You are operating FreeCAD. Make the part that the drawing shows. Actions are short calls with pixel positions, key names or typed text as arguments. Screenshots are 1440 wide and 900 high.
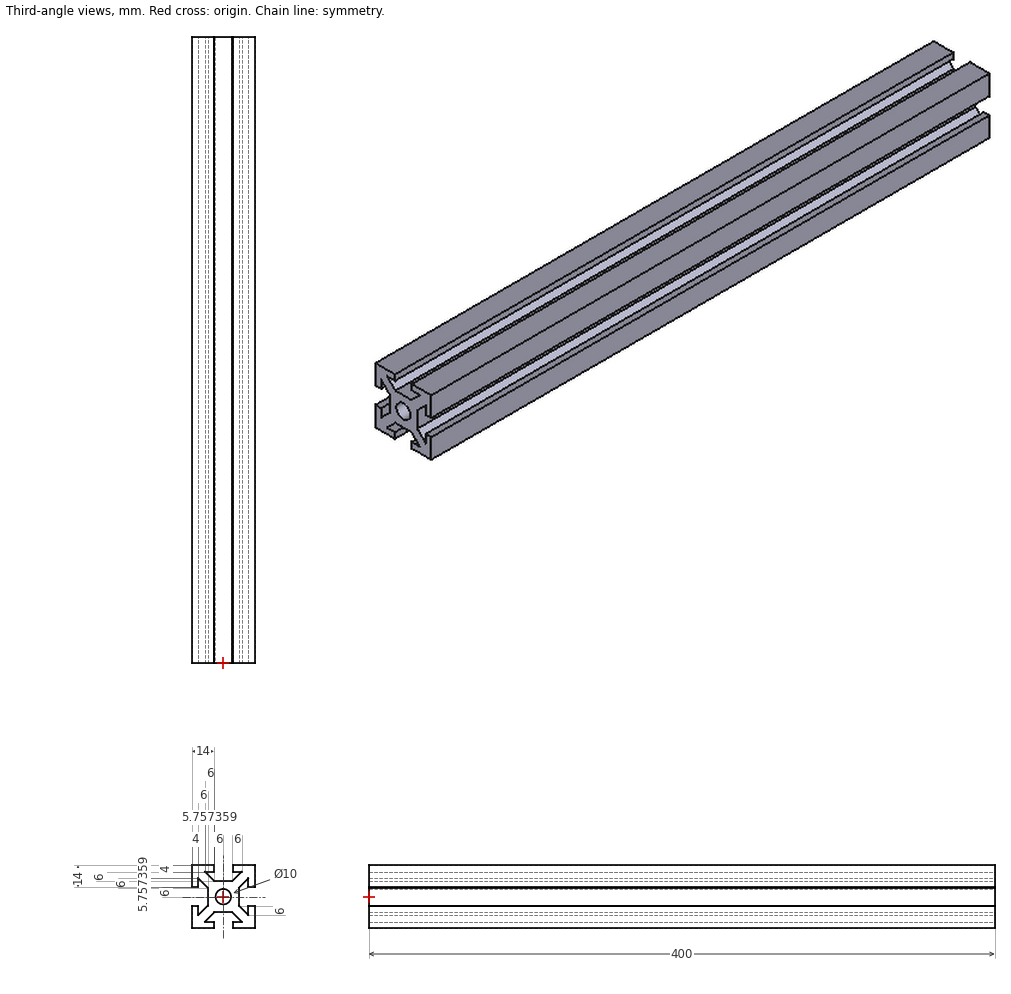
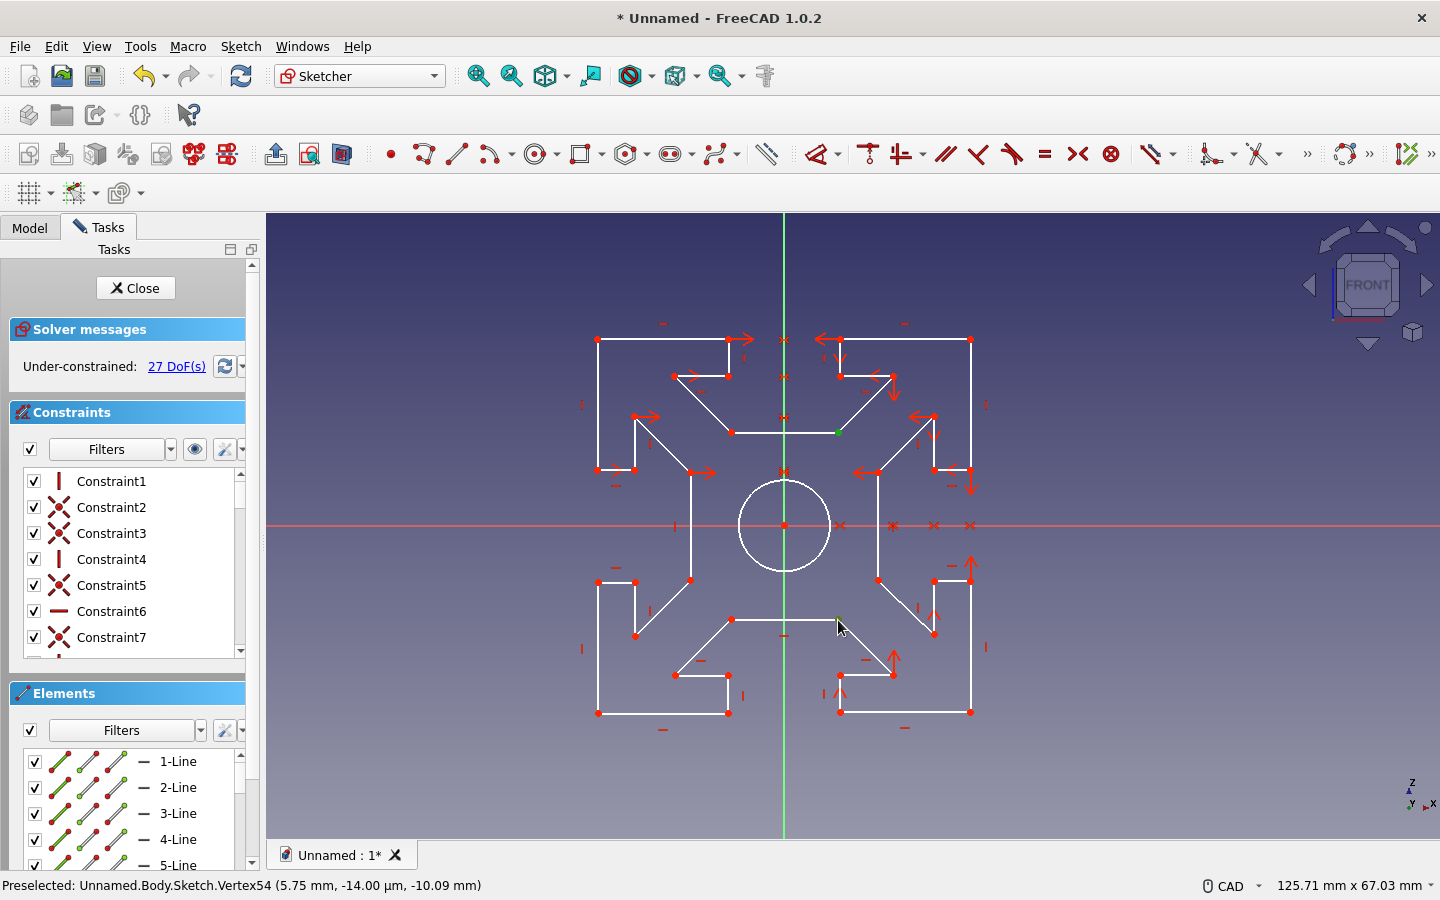
click(364, 526)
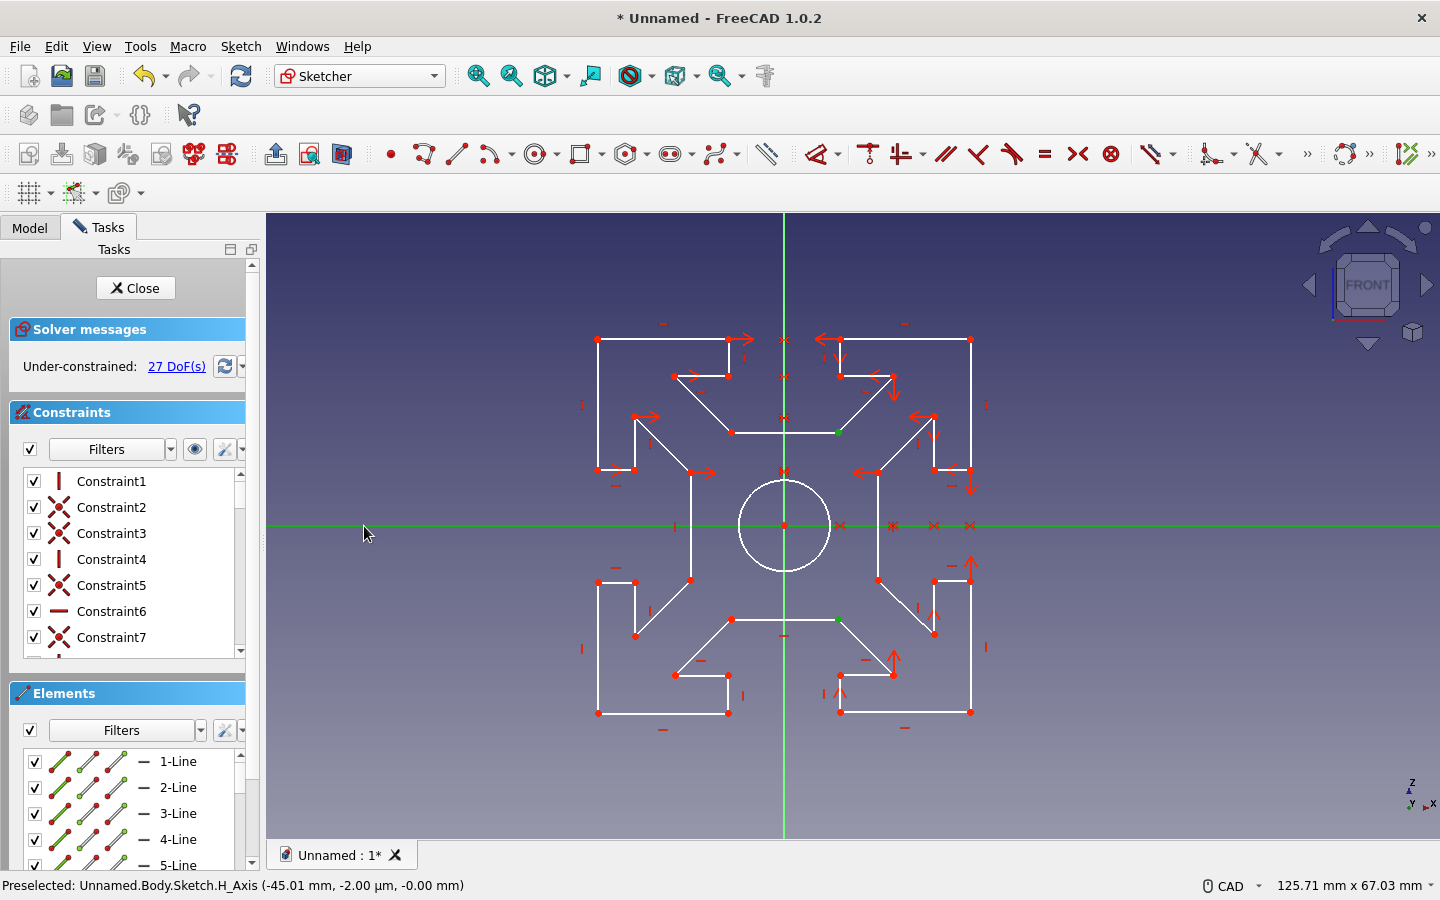
key(s)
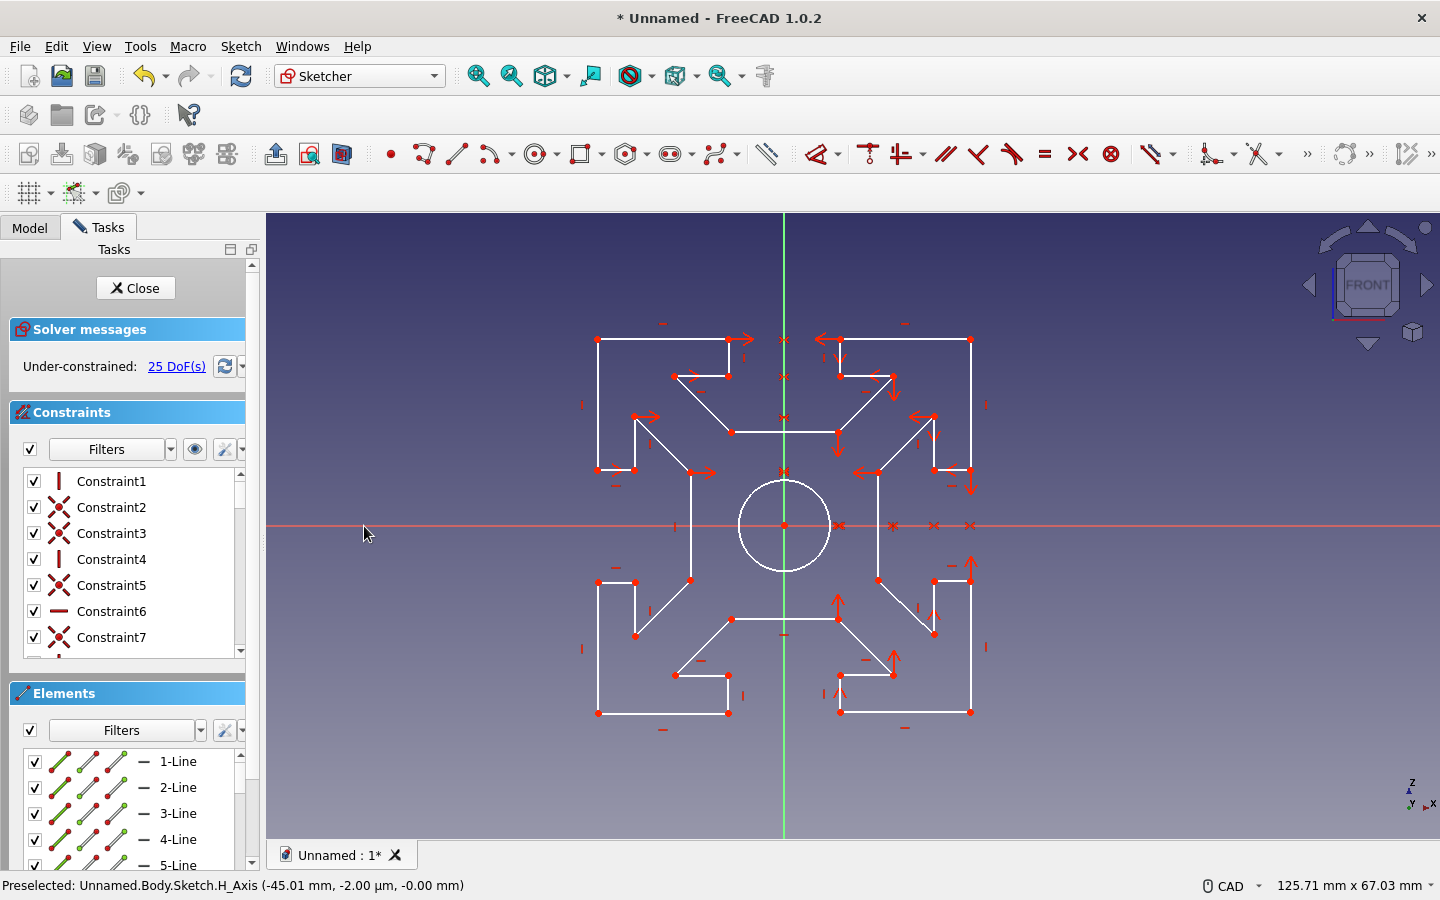
click(675, 376)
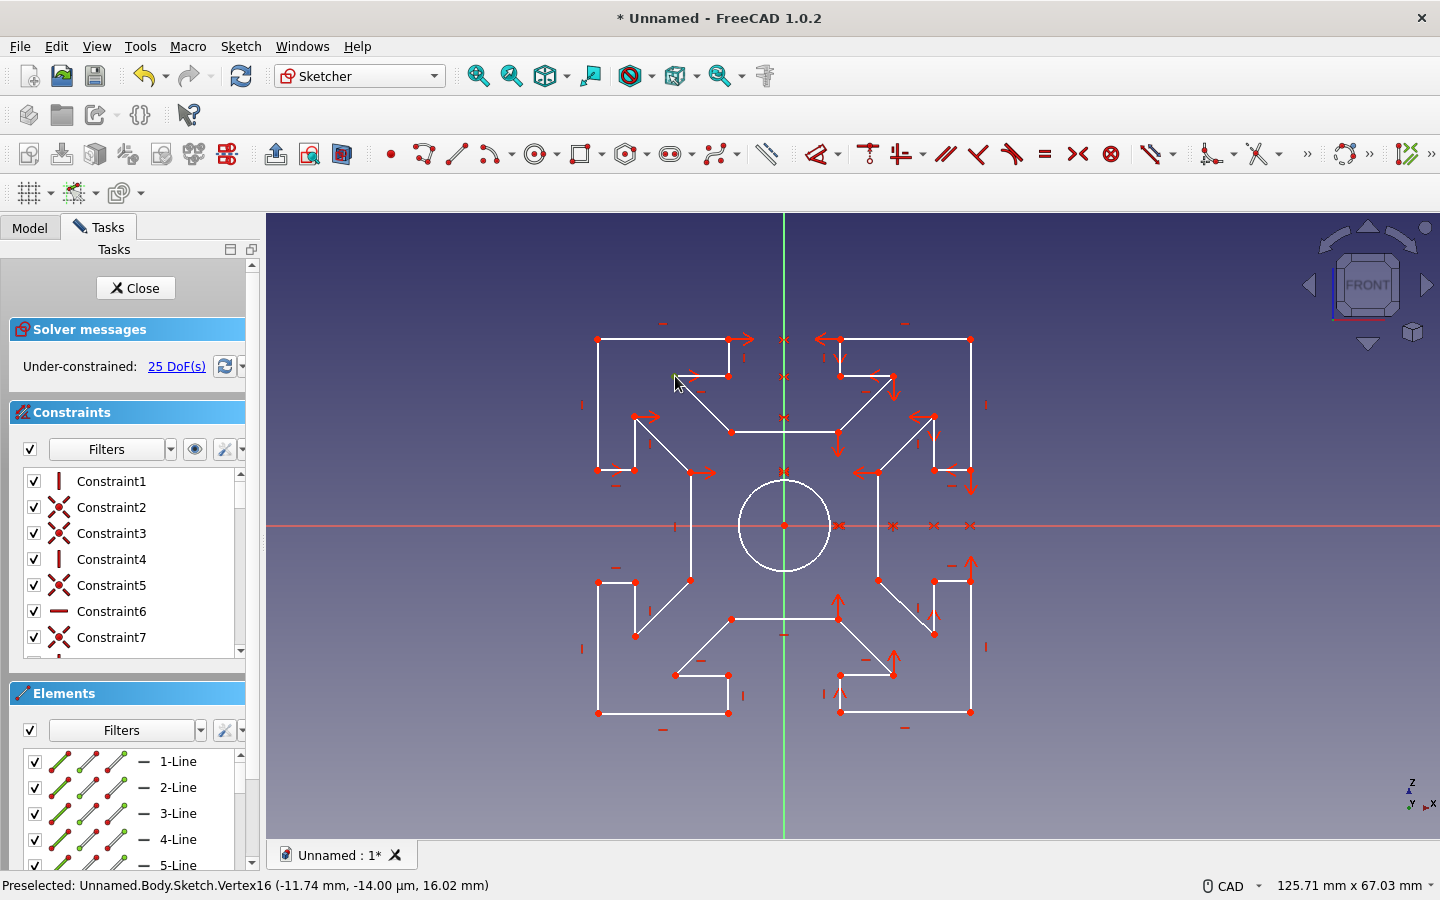
click(675, 676)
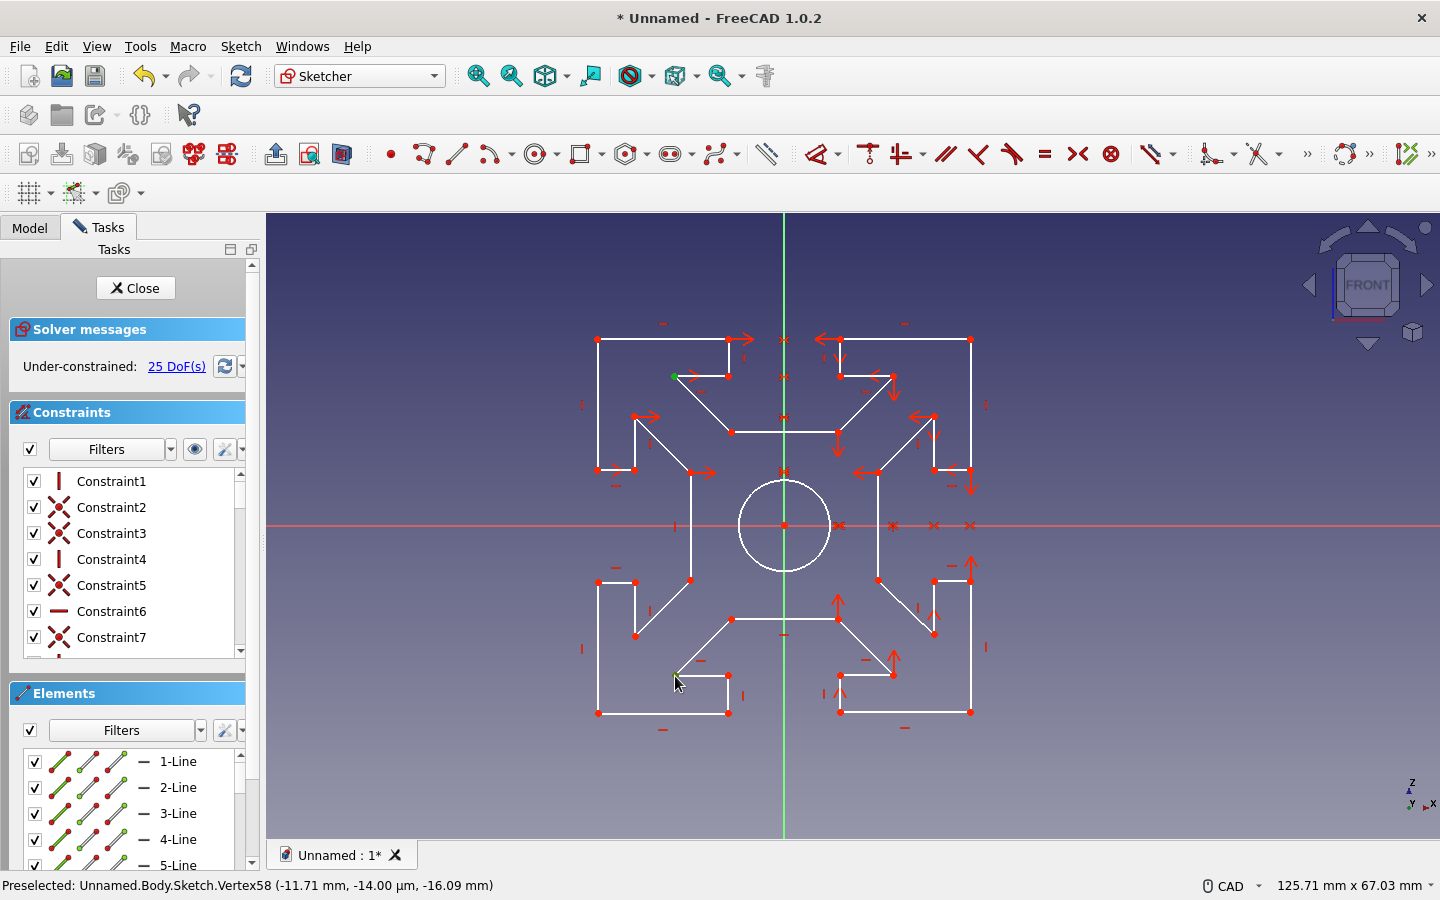
click(364, 526)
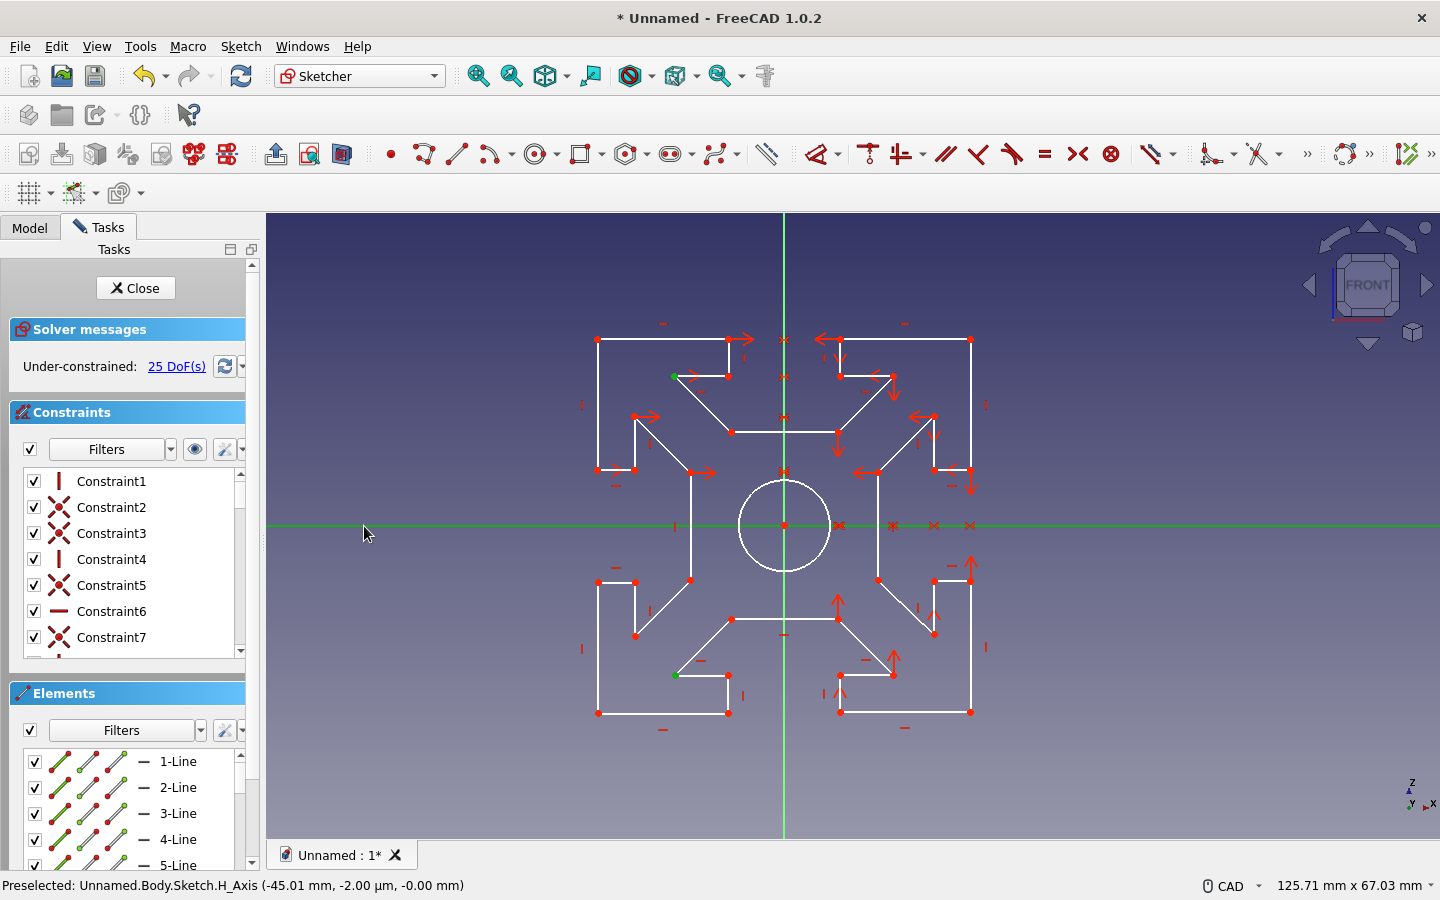
key(s)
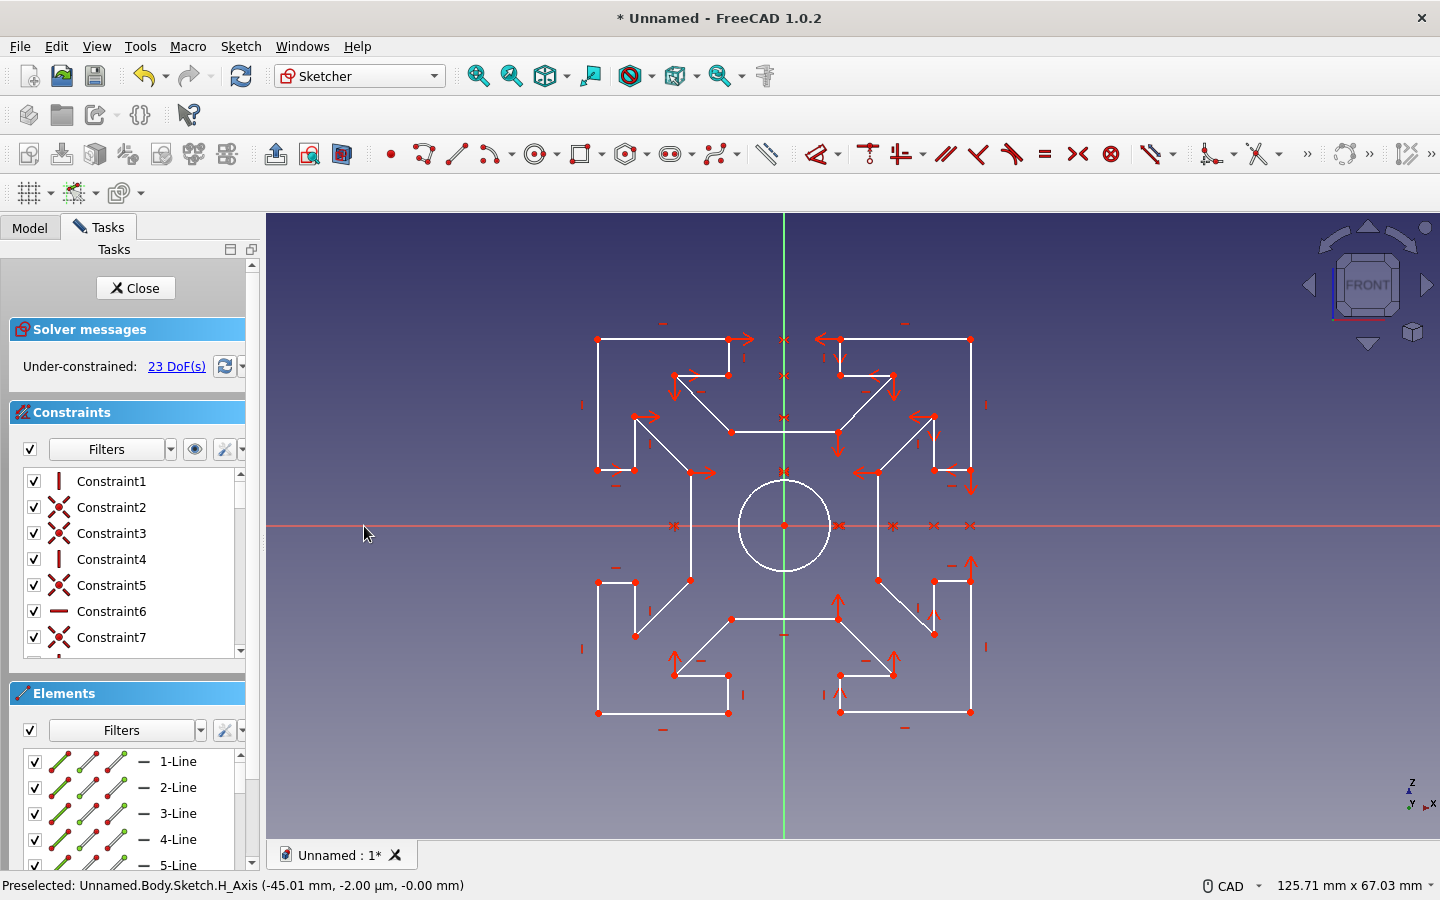
click(729, 339)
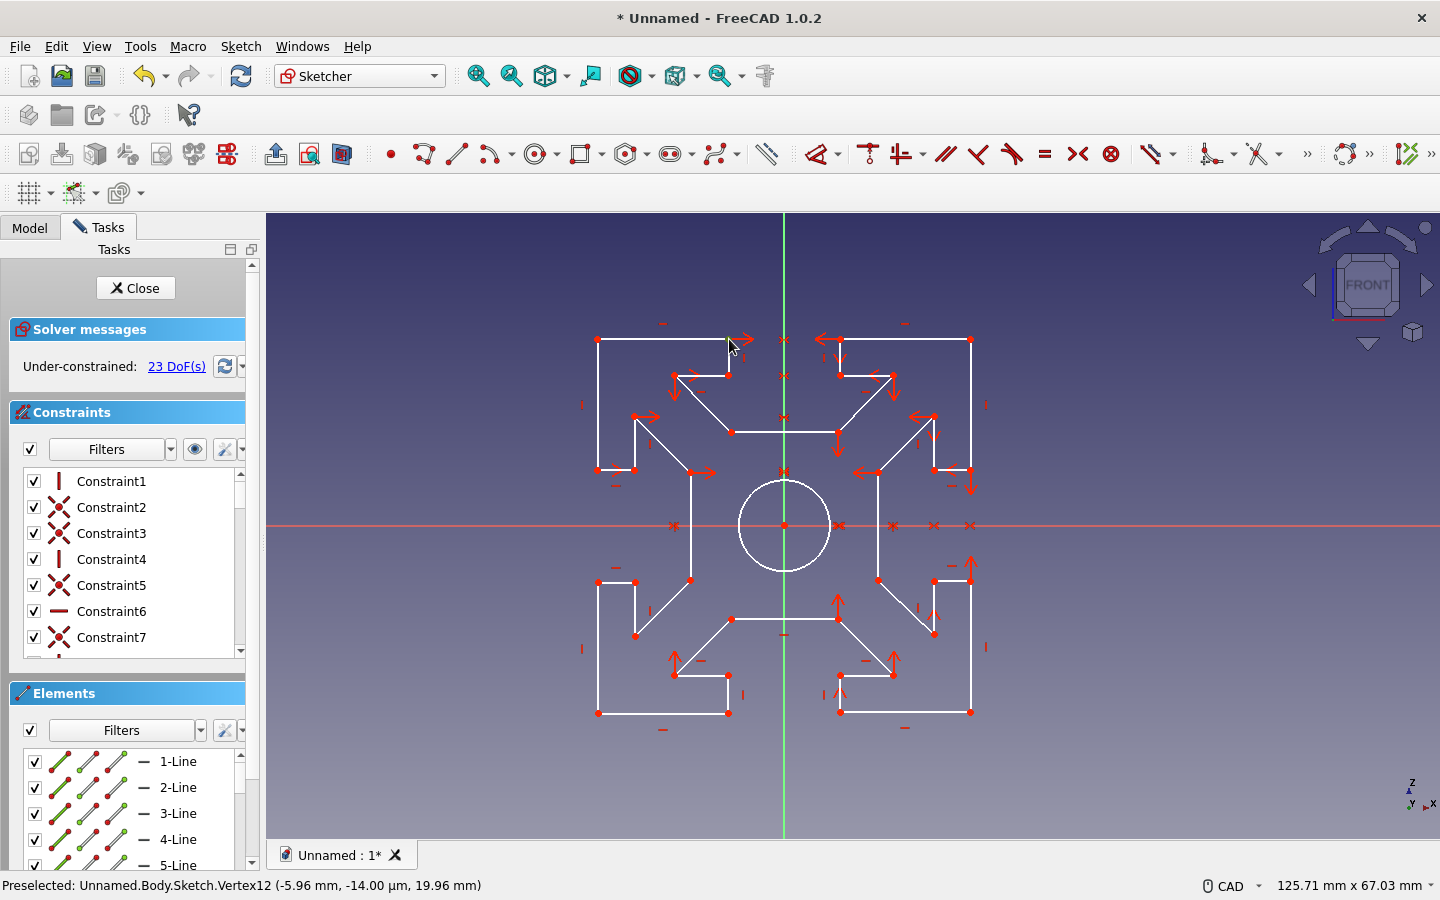
click(728, 714)